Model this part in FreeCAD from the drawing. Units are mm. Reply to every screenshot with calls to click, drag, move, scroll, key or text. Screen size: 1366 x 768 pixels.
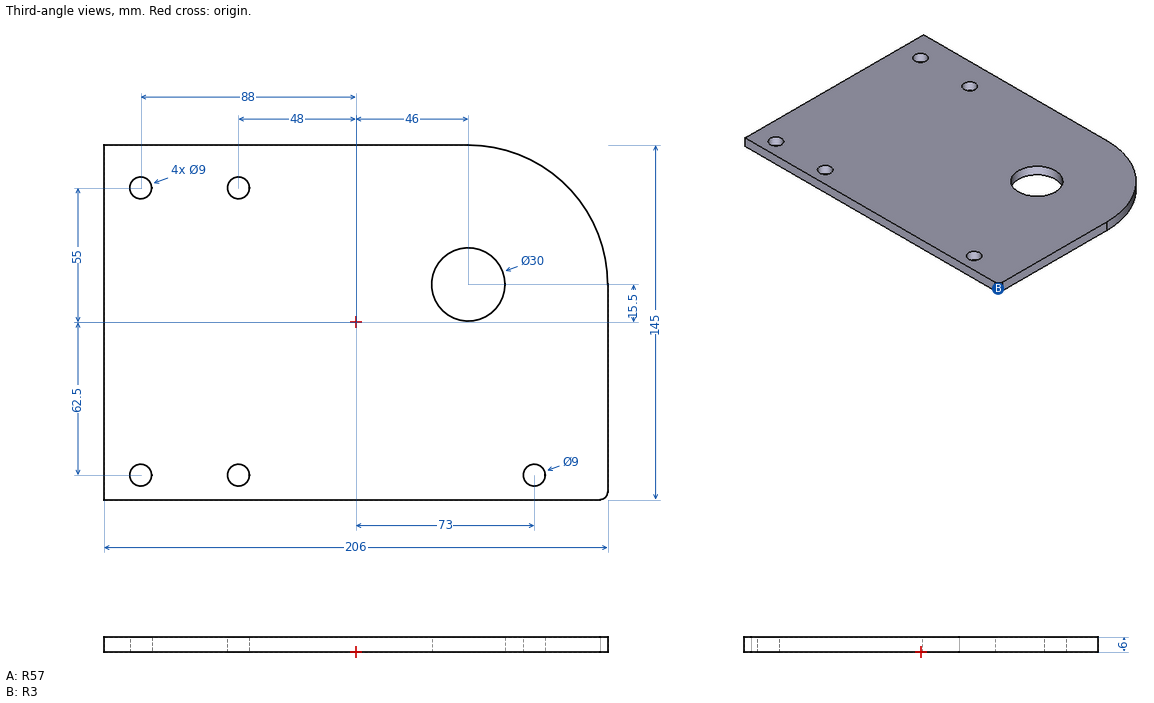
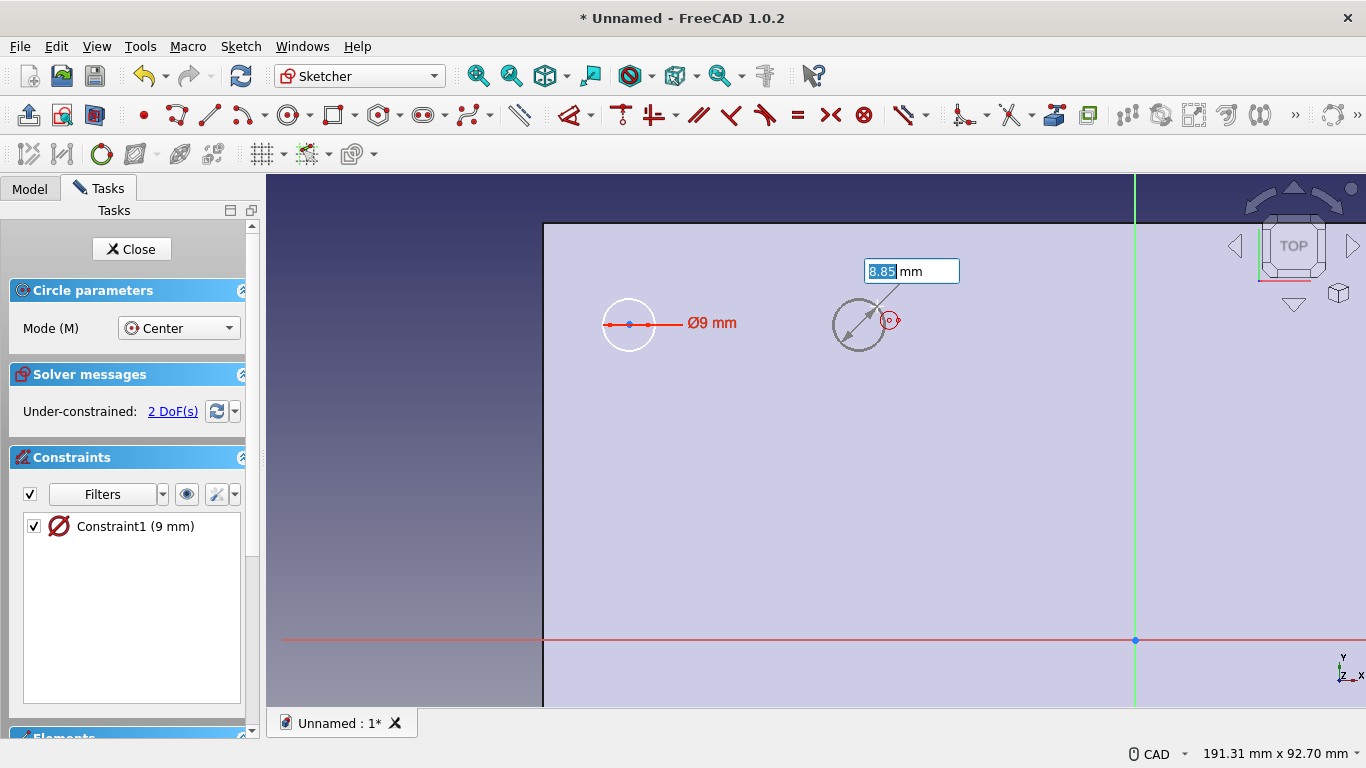
text(9)
key(Return)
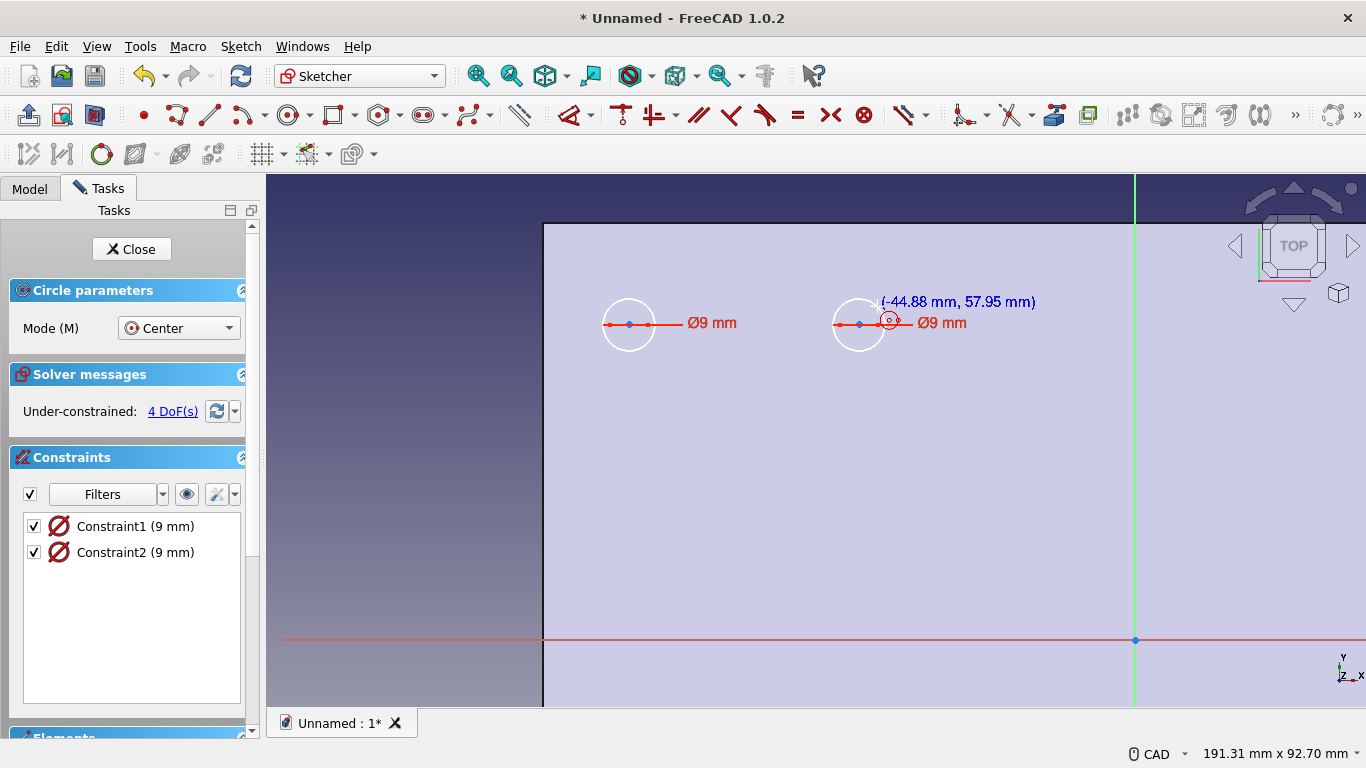
scroll(648, 260, down, 4)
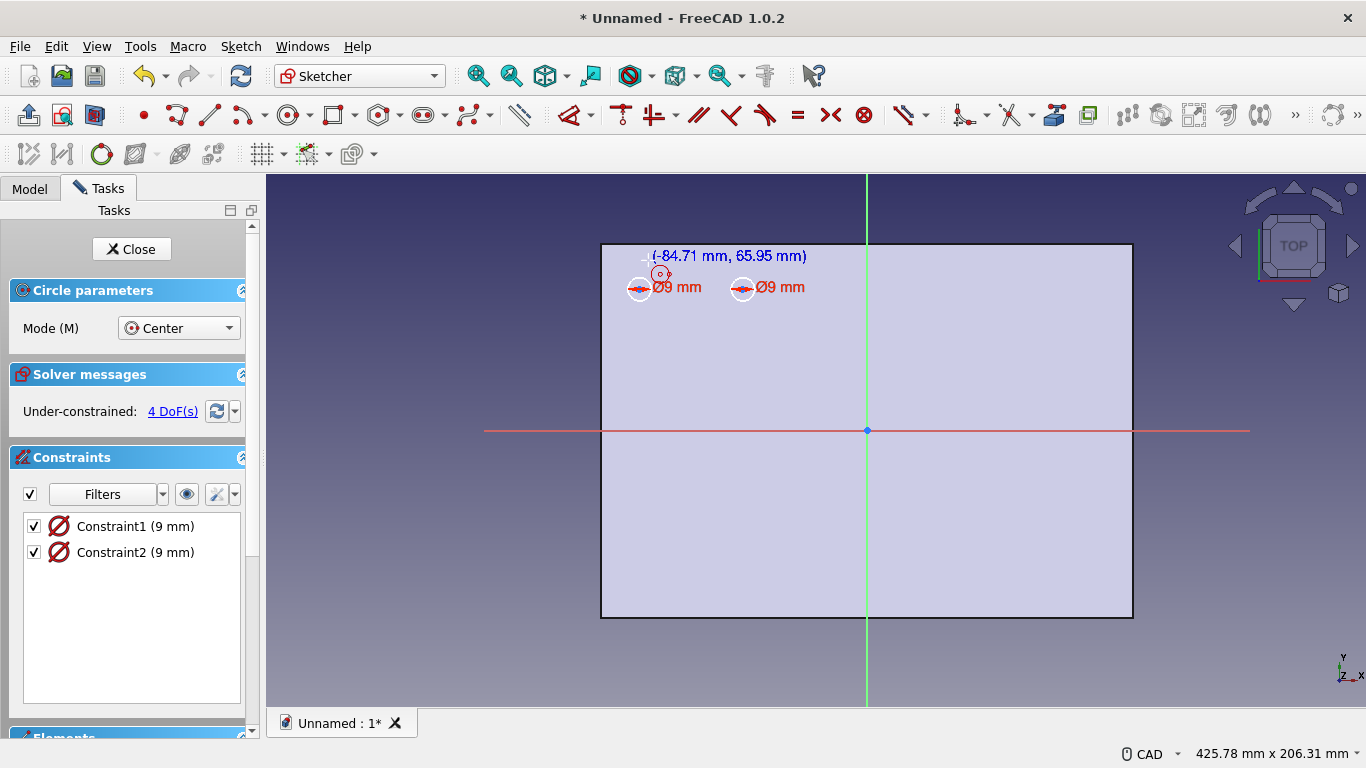
scroll(640, 592, up, 4)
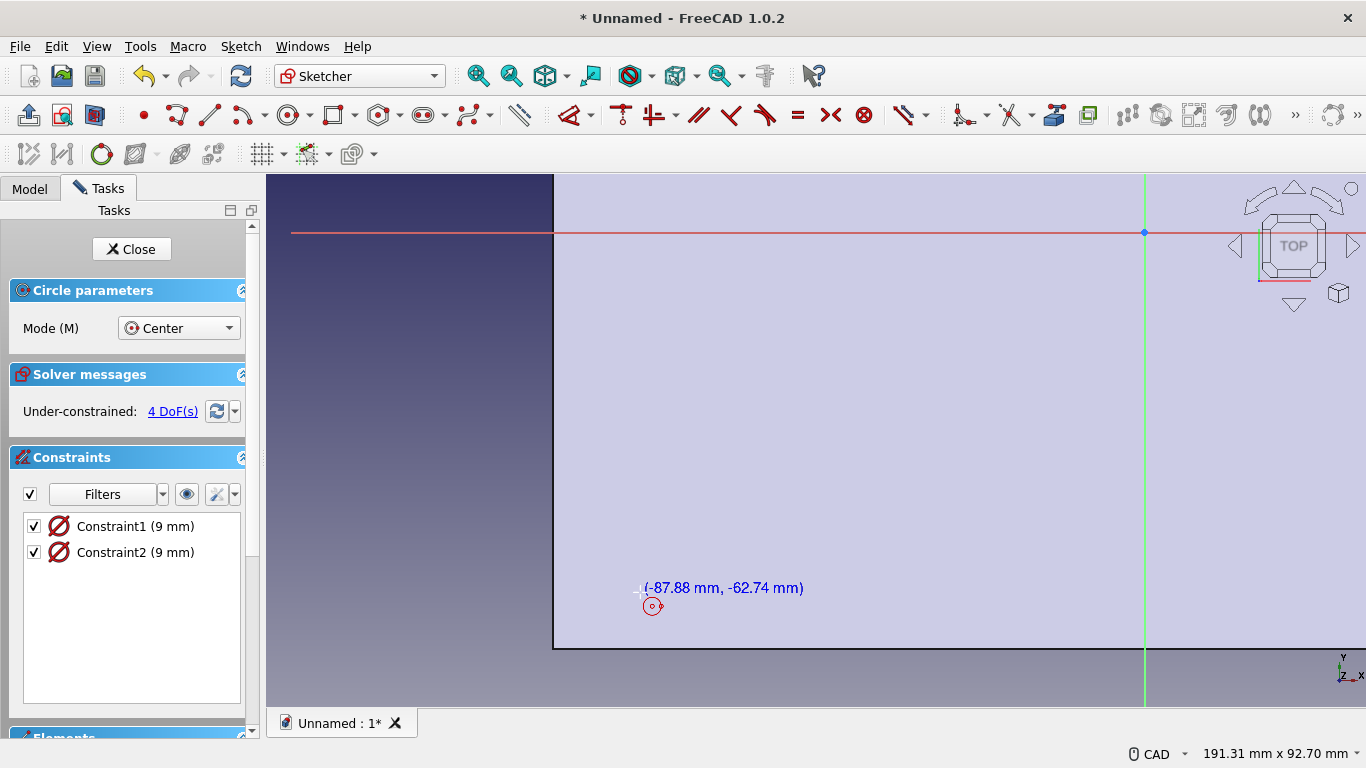
click(639, 592)
move(657, 574)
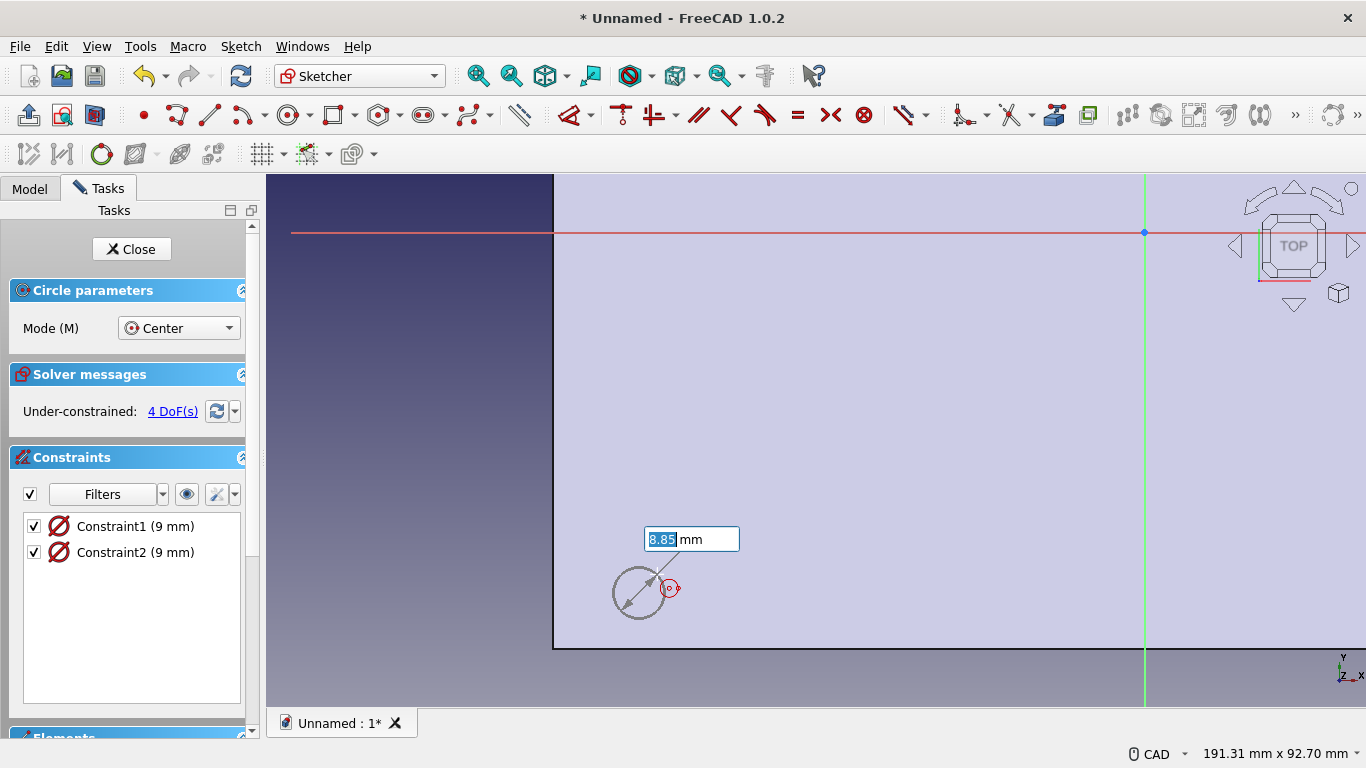
text(9)
key(Return)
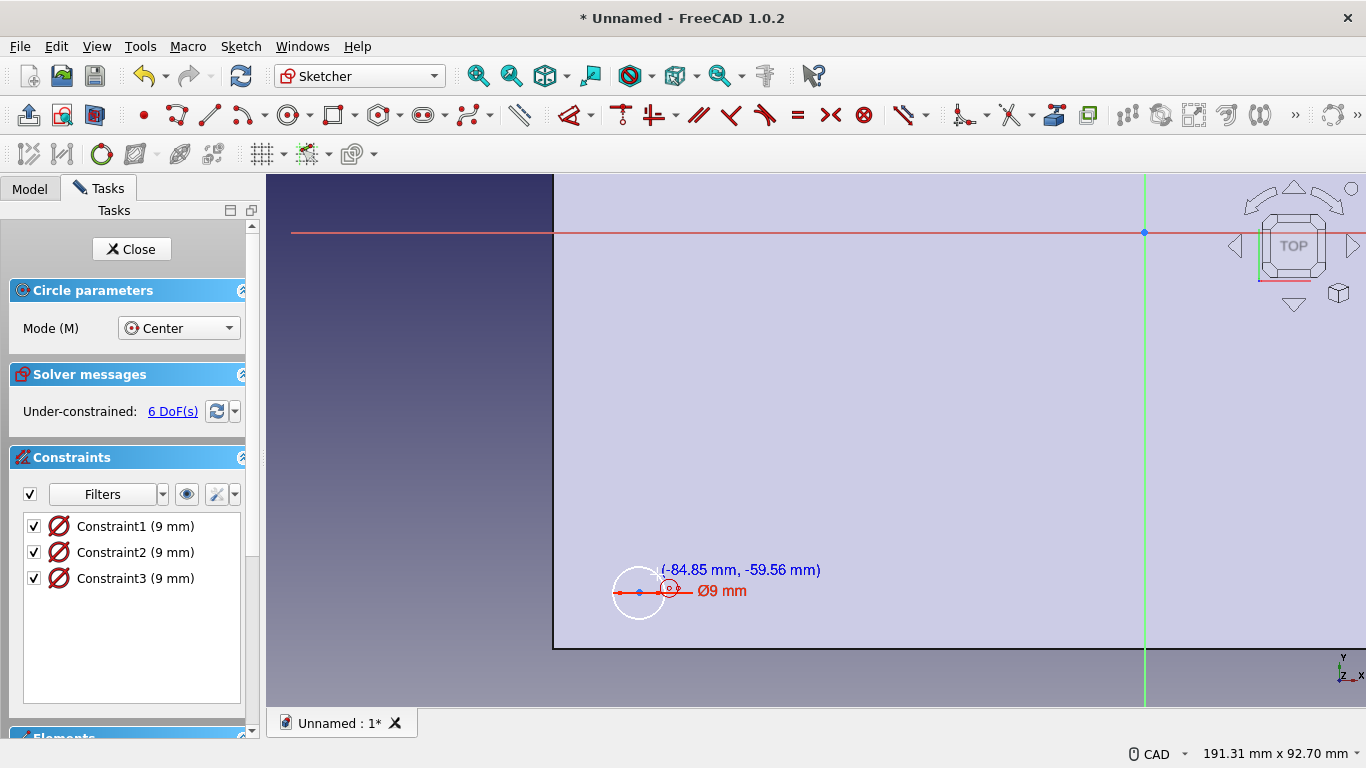
click(869, 592)
move(887, 574)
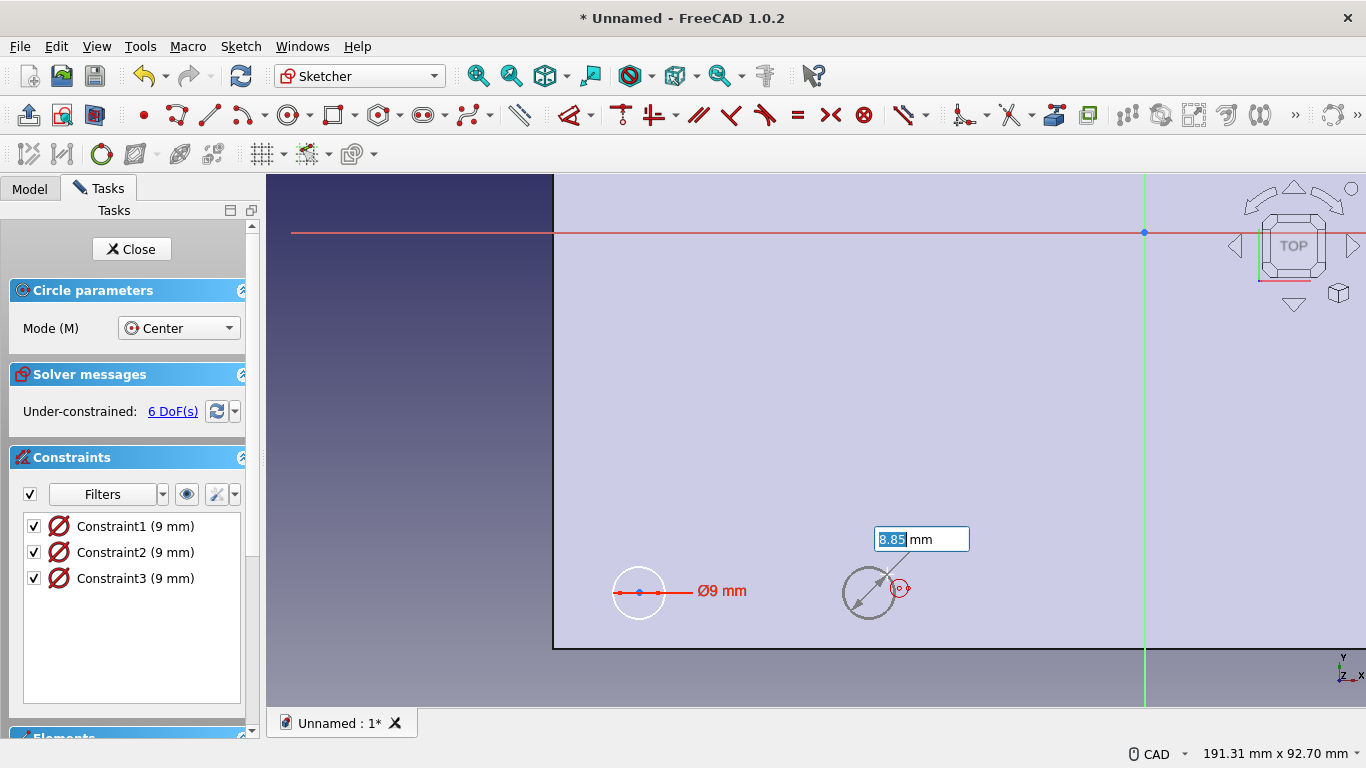
text(9)
key(Return)
key(Escape)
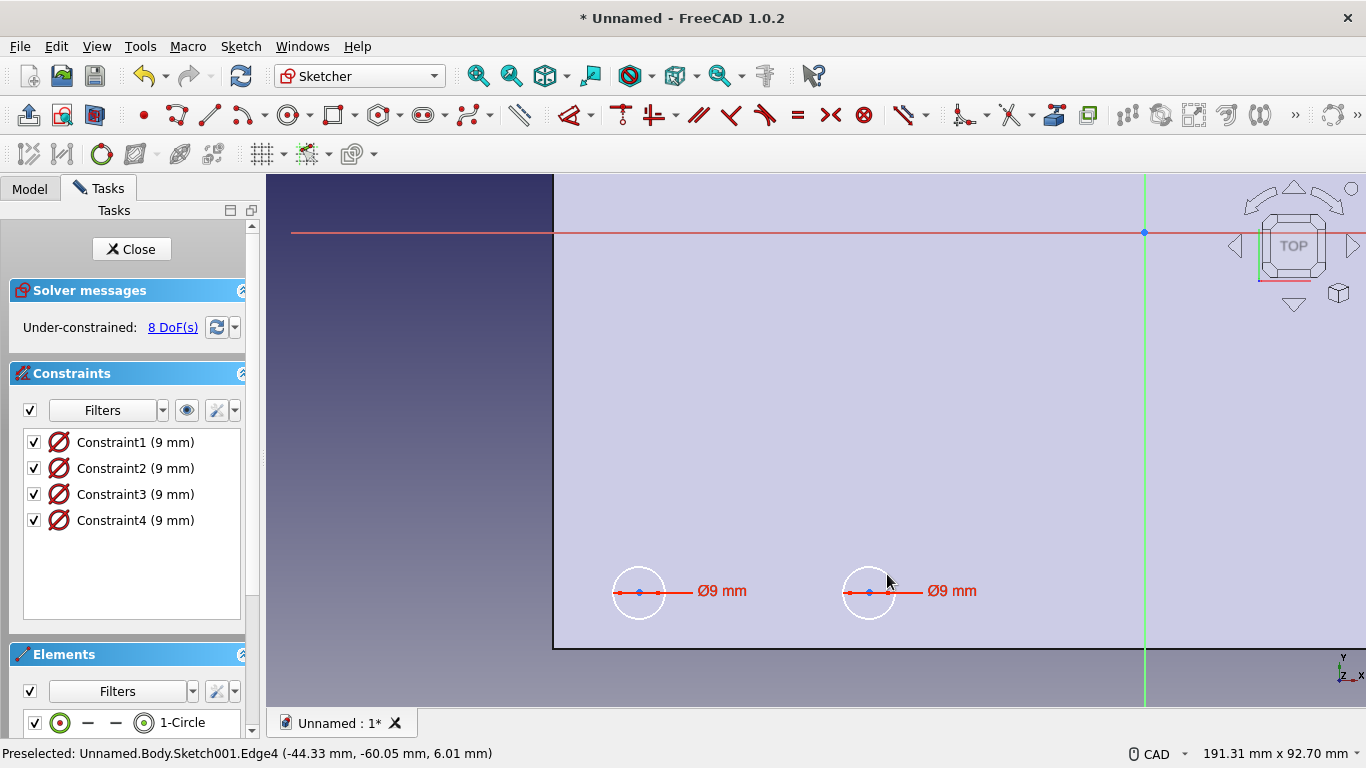
scroll(640, 593, down, 4)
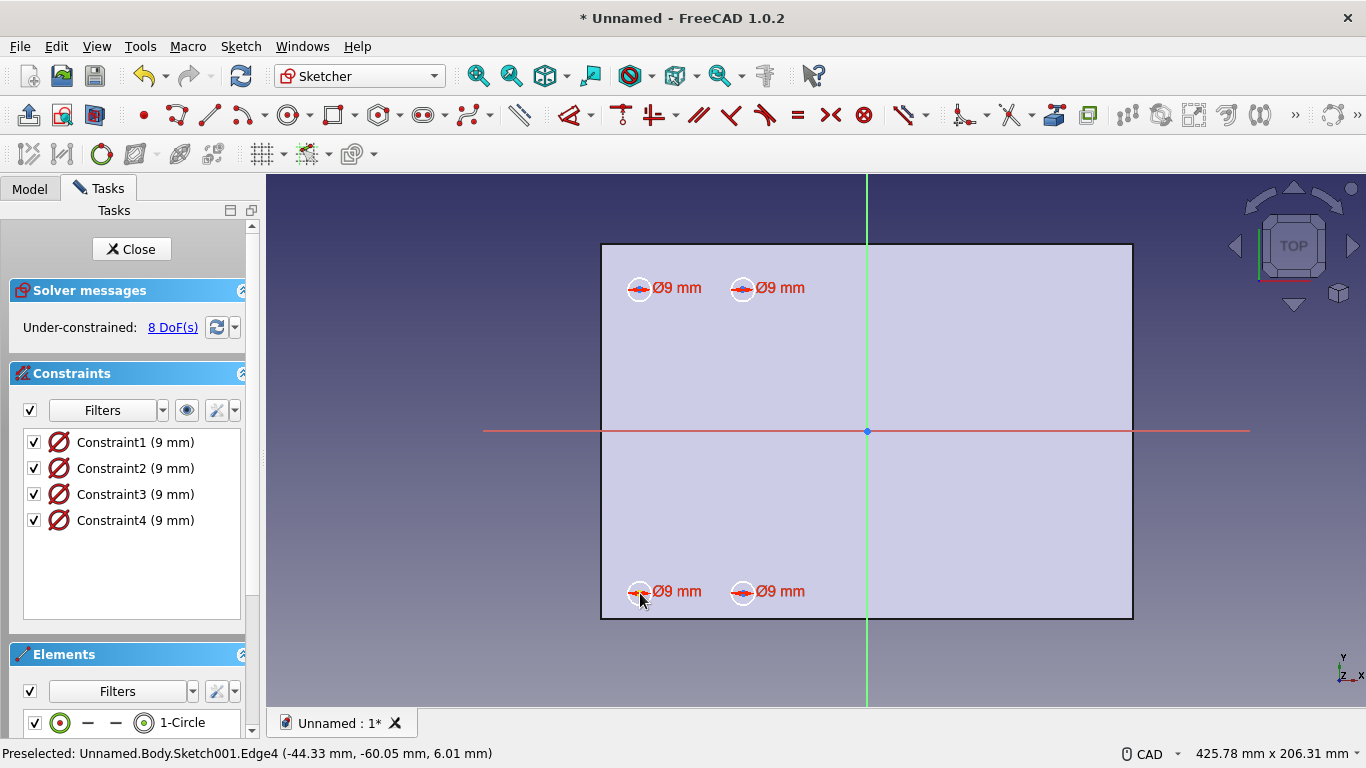
click(640, 290)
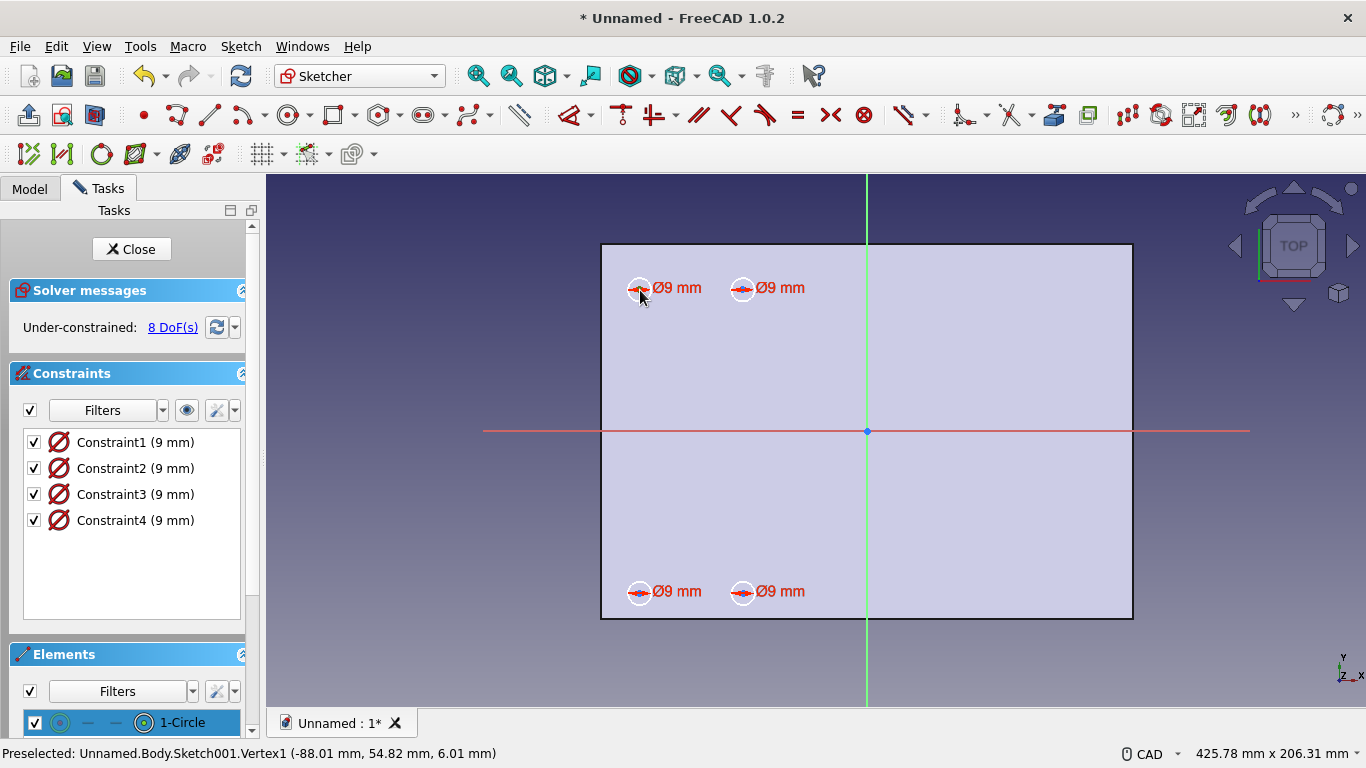
key(l)